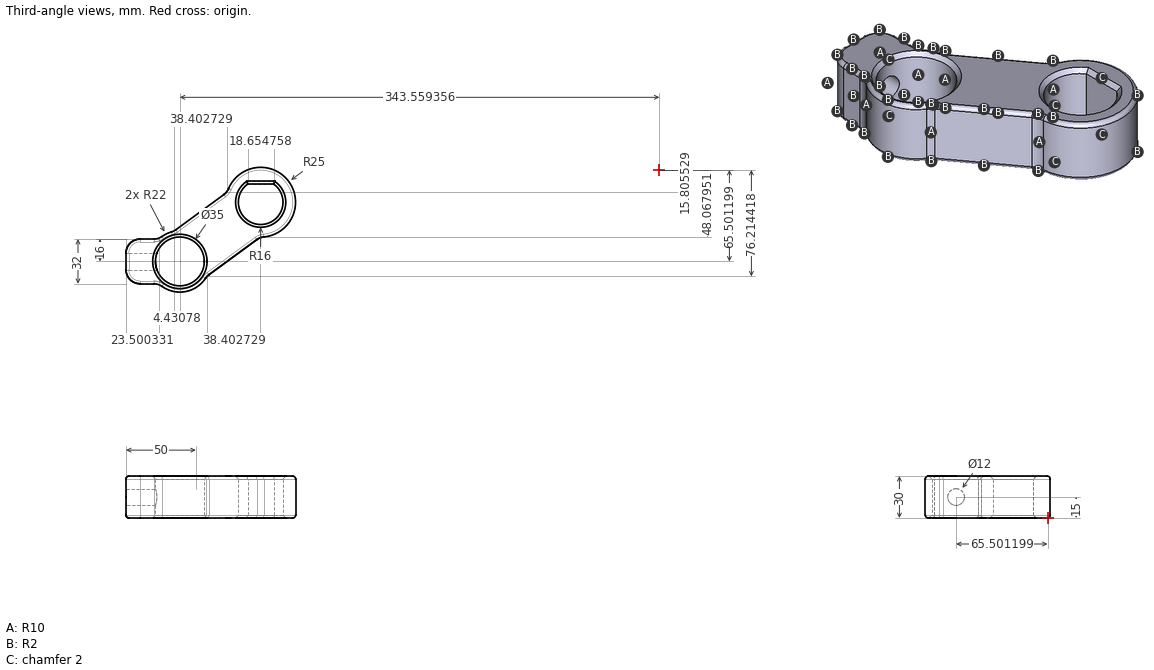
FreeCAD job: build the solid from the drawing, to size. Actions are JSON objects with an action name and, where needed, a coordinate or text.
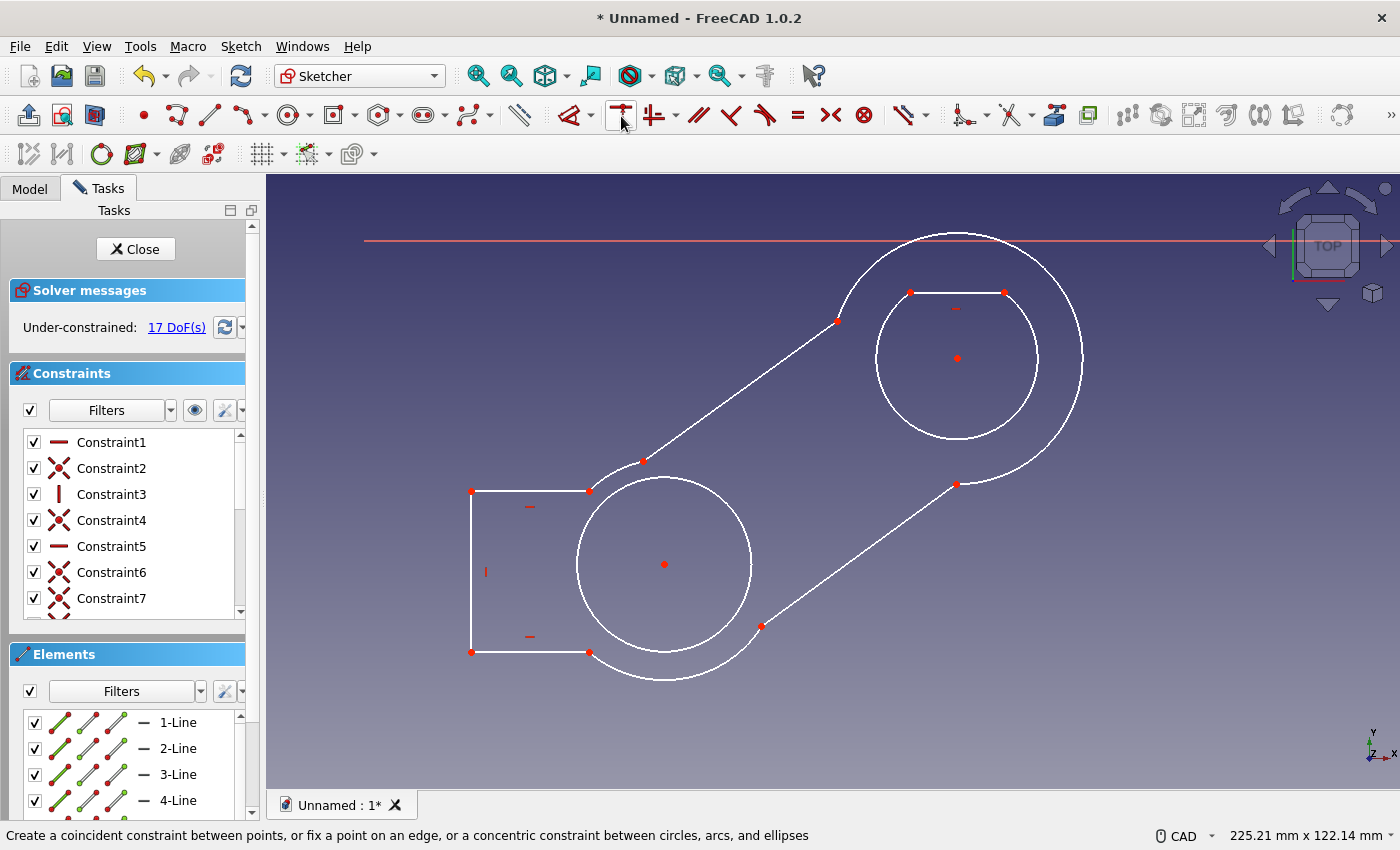
{"action": "left_click", "coordinate": [625, 467]}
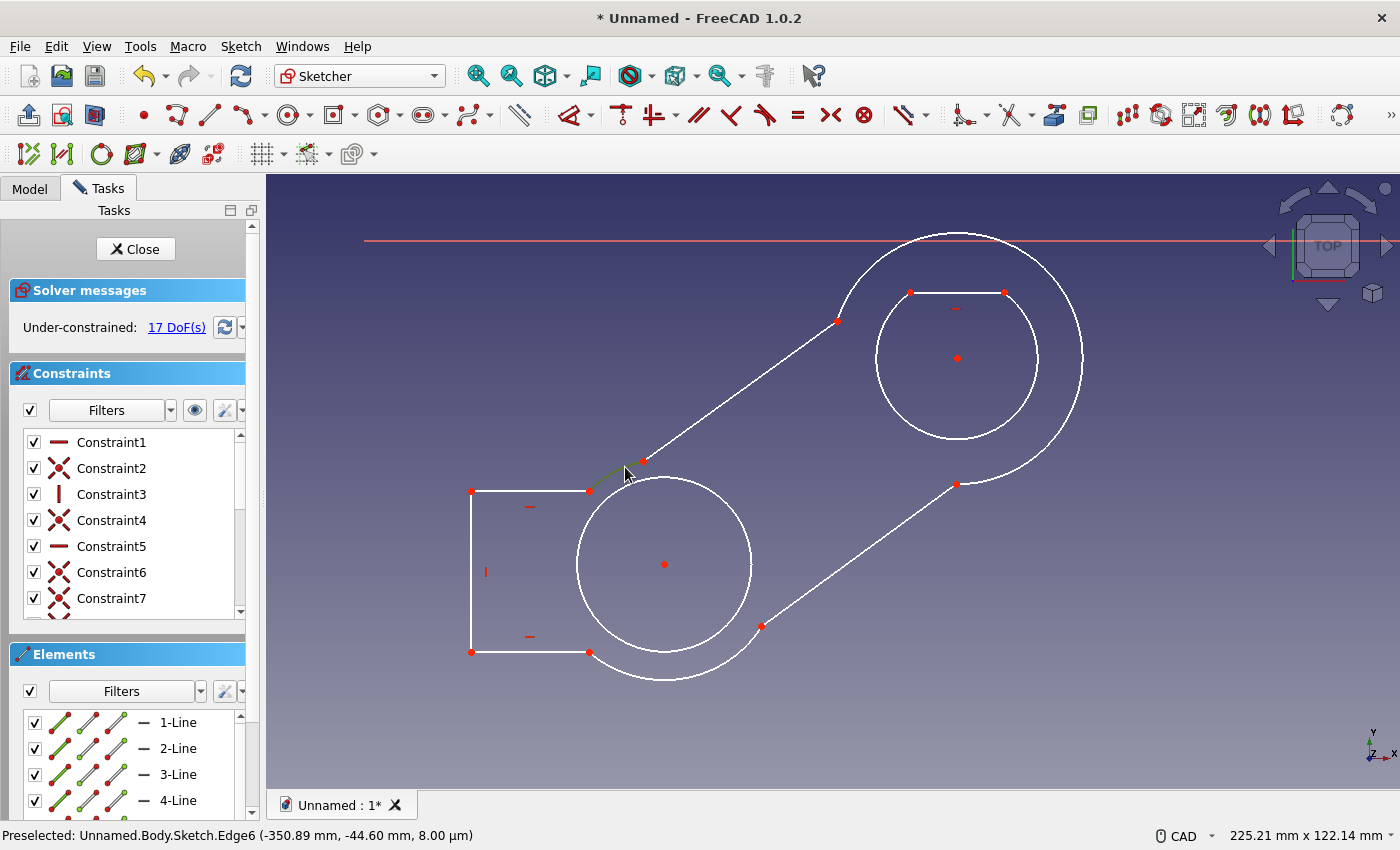
{"action": "left_click", "coordinate": [642, 678]}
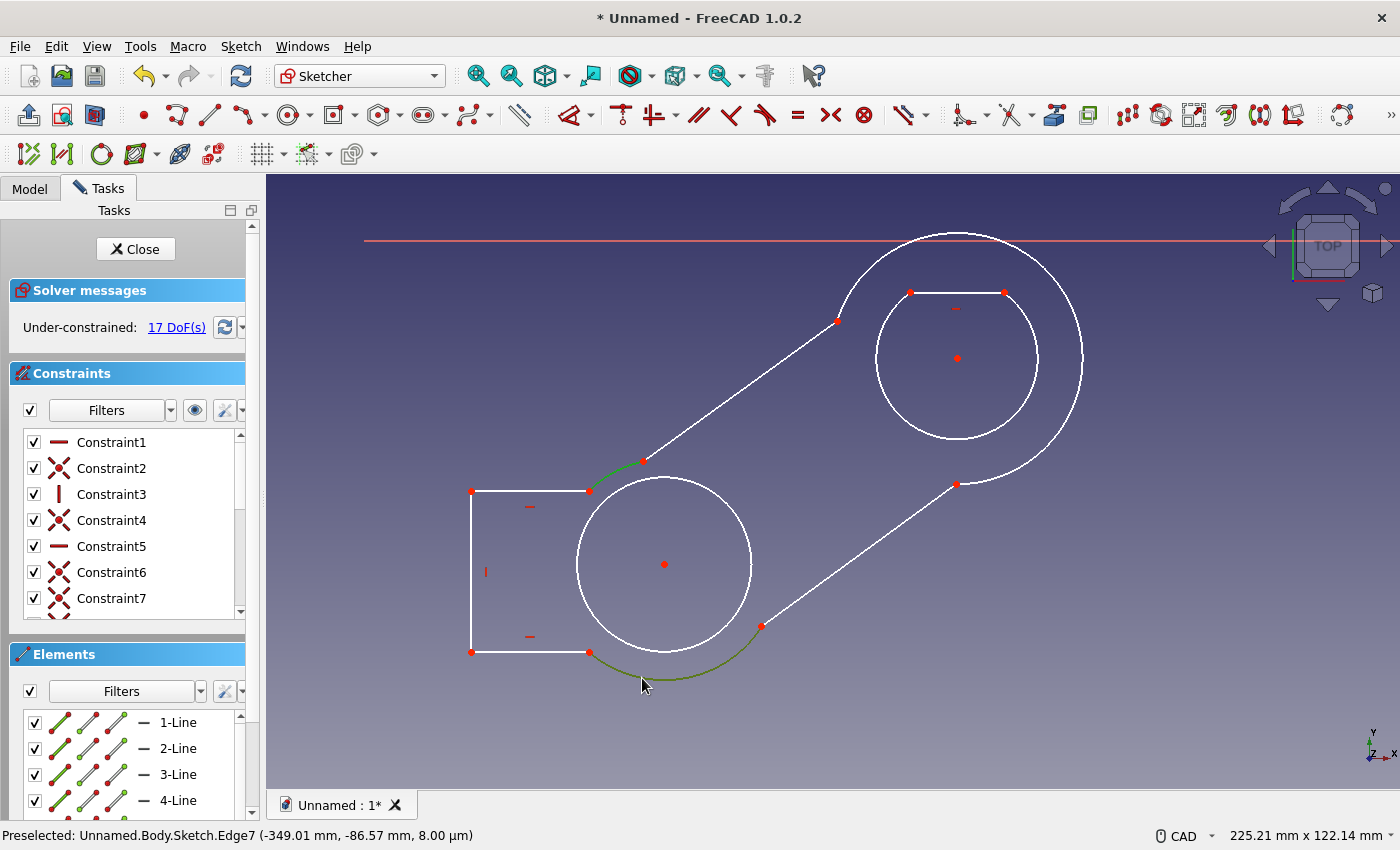
{"action": "left_click", "coordinate": [798, 116]}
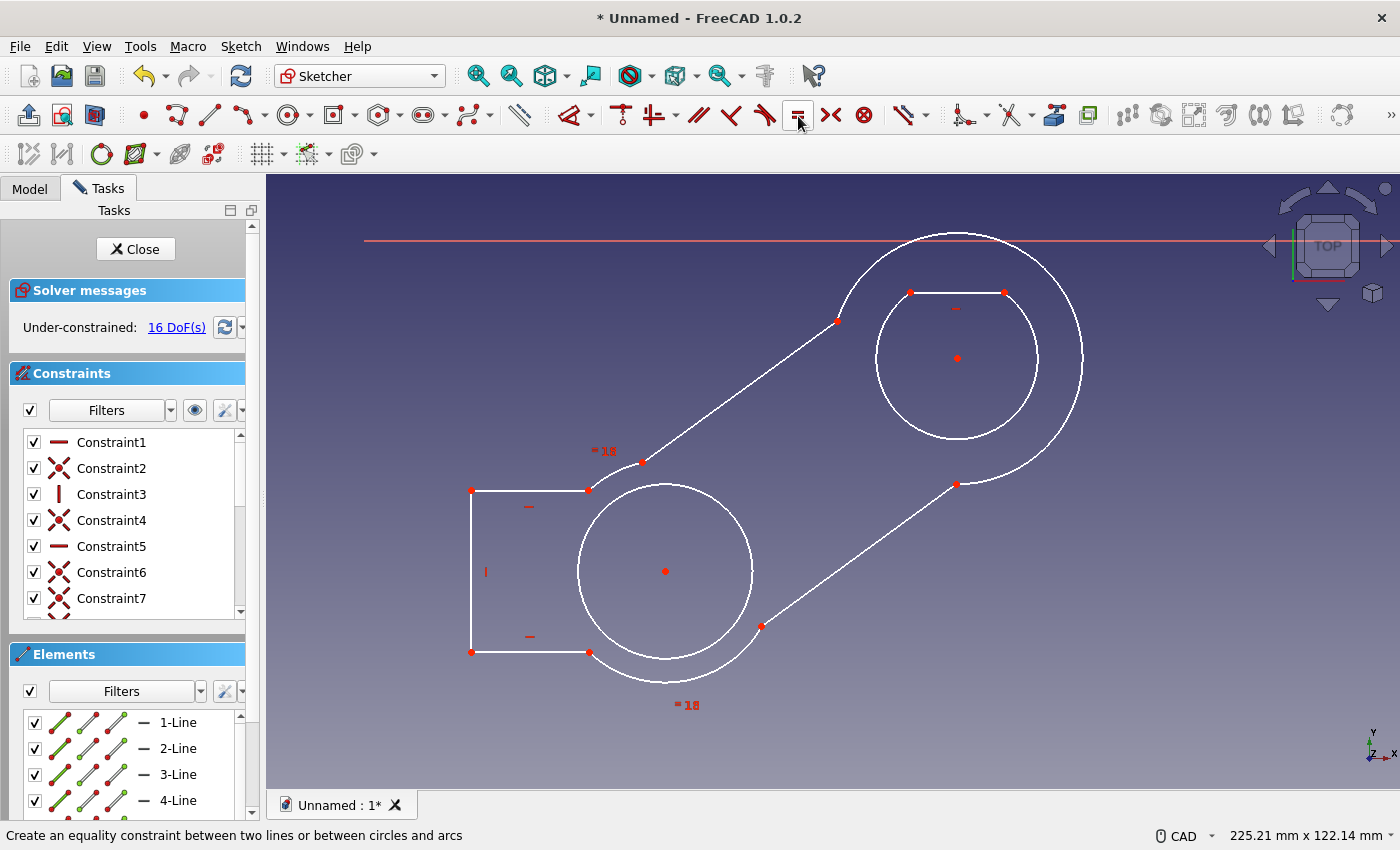
{"action": "left_click", "coordinate": [625, 468]}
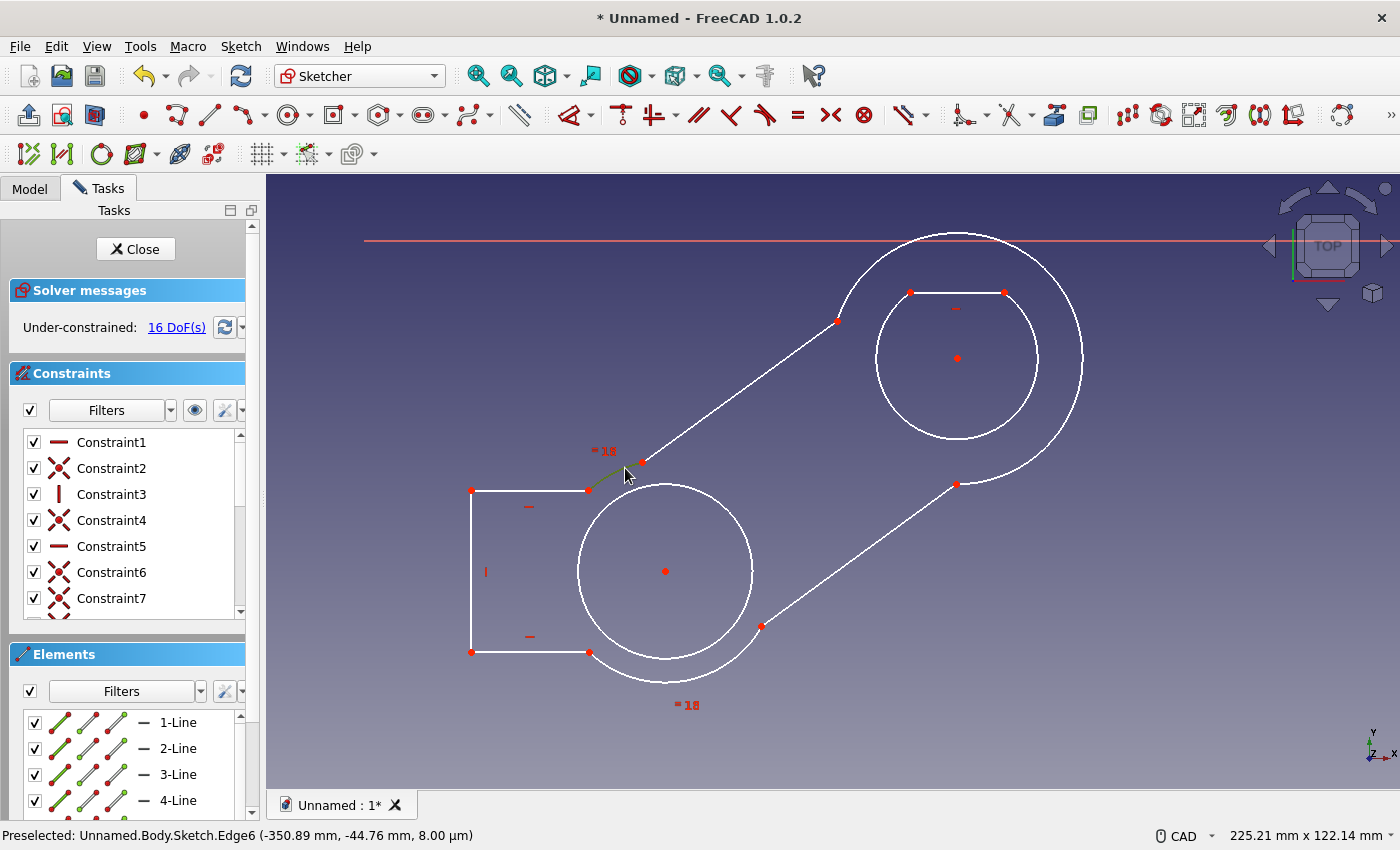
{"action": "key", "text": "k r"}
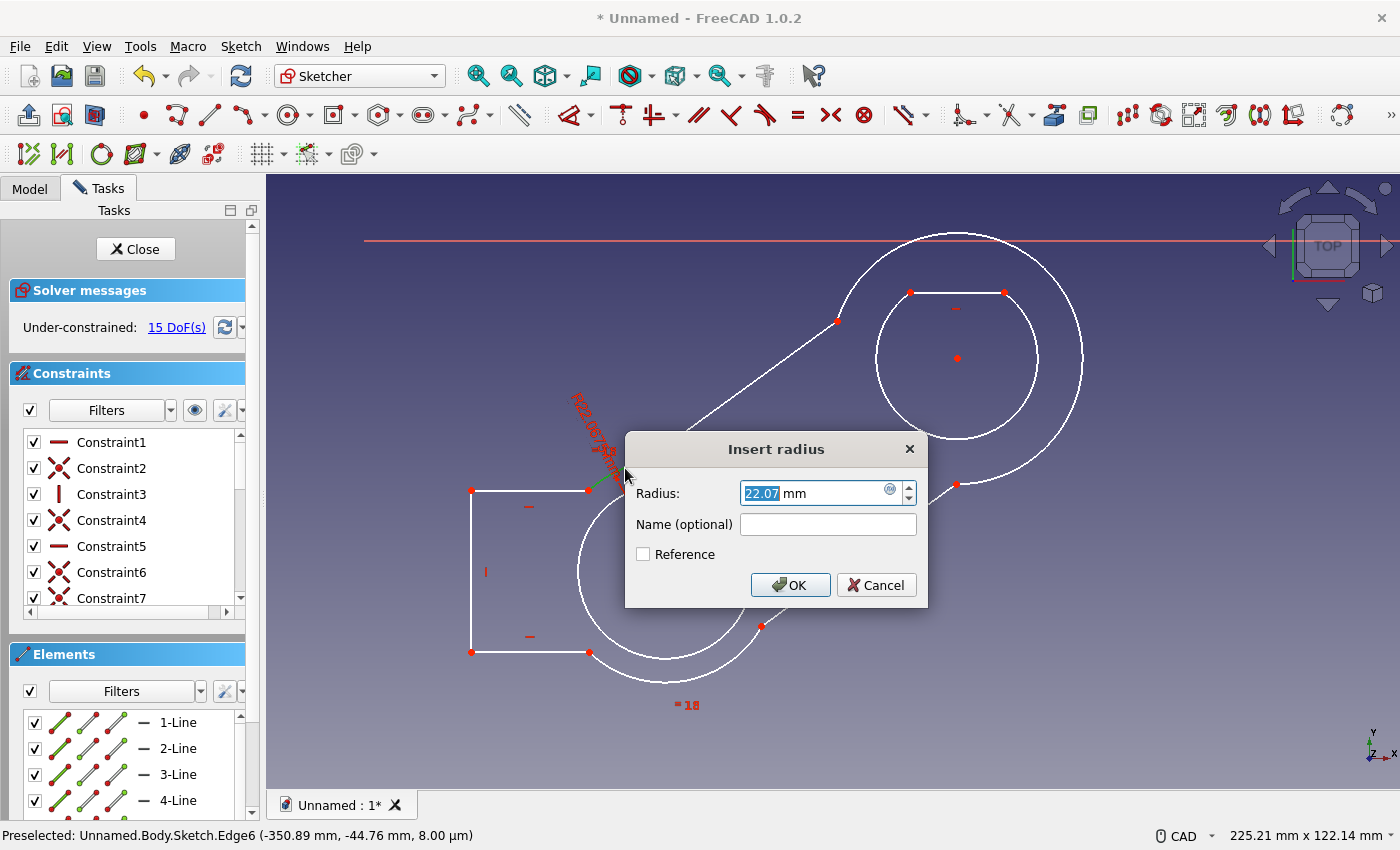
{"action": "type", "text": "22"}
{"action": "key", "text": "Return"}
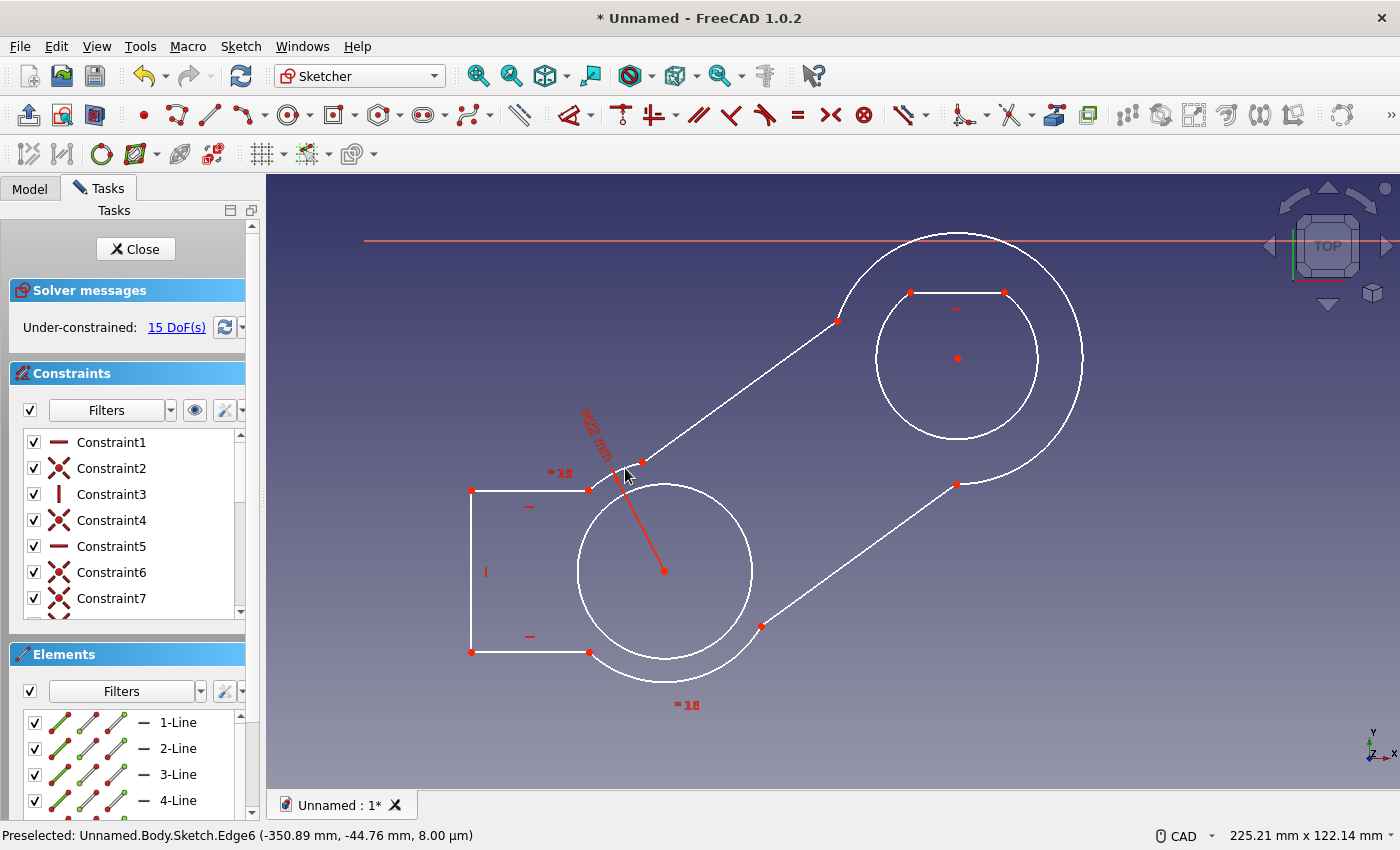
{"action": "left_click", "coordinate": [1079, 390]}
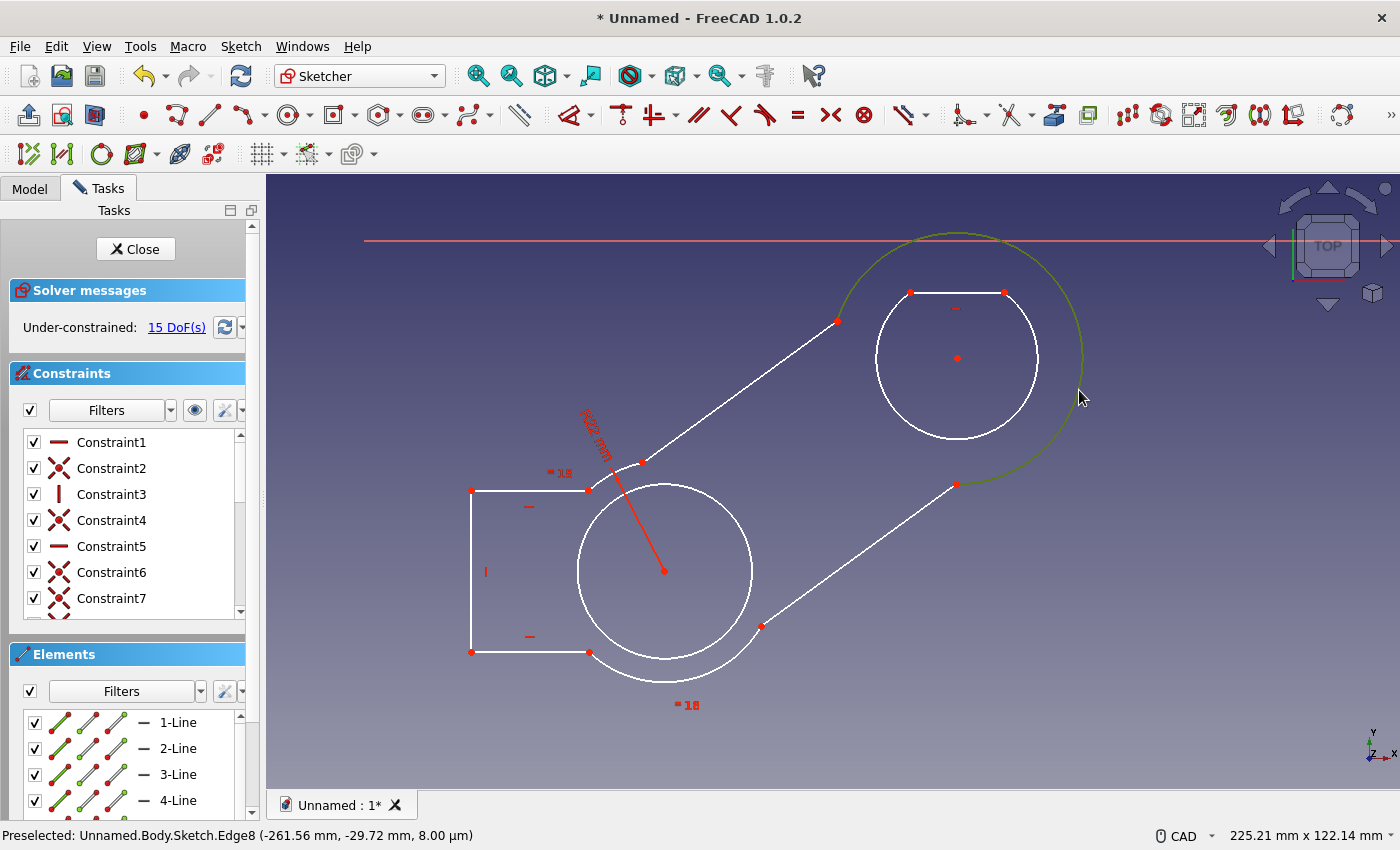
{"action": "left_click", "coordinate": [590, 116]}